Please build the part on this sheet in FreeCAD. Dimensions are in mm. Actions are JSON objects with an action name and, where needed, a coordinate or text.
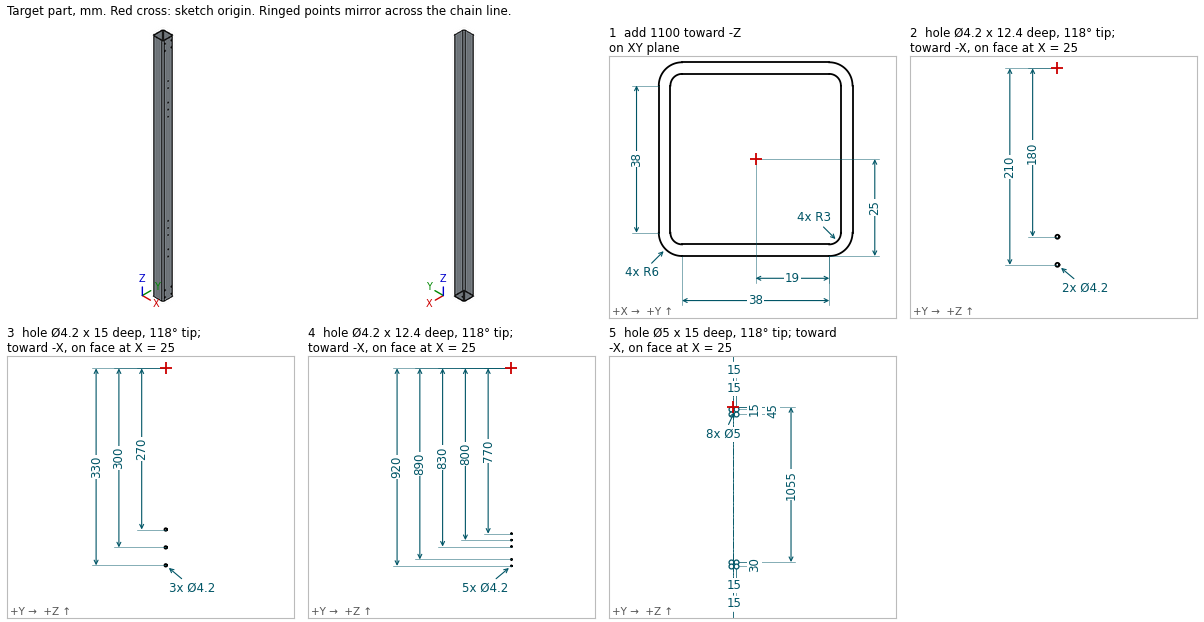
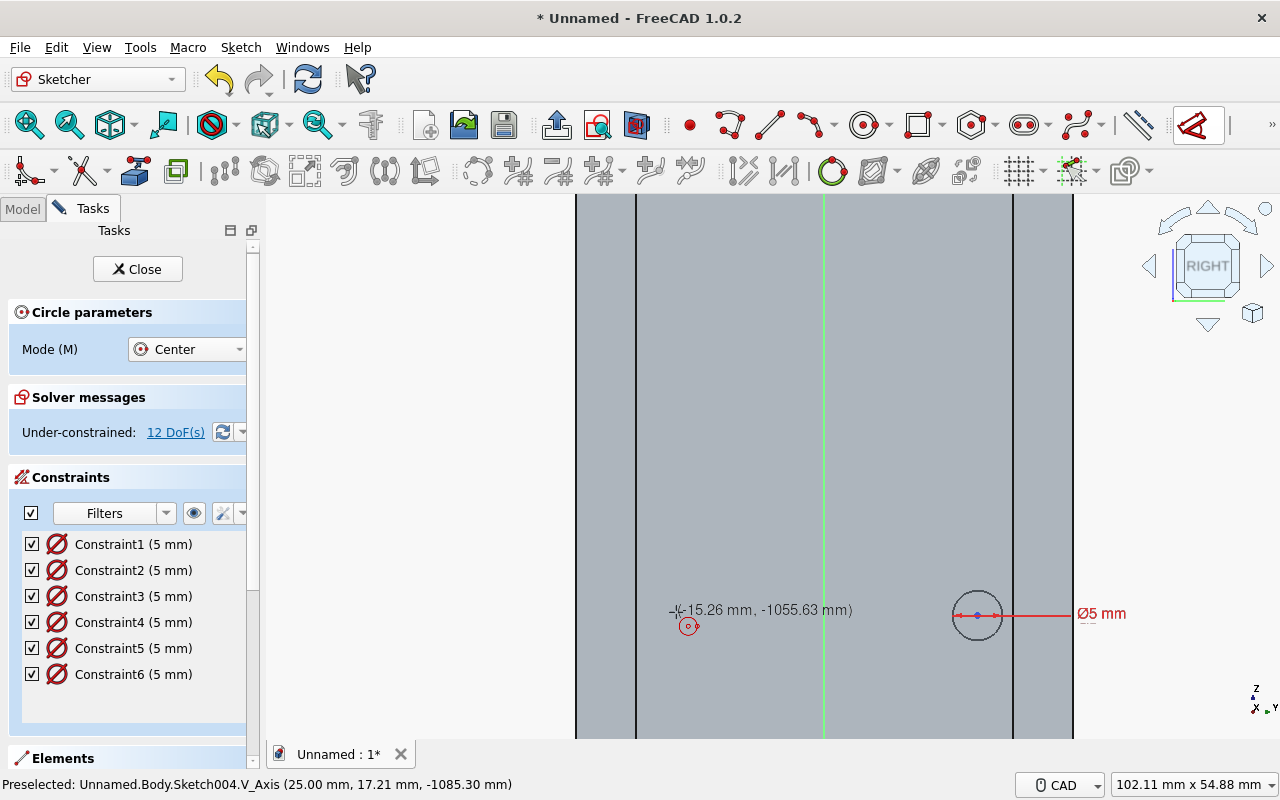
{"action": "scroll", "coordinate": [700, 637], "scroll_direction": "down", "scroll_amount": 17}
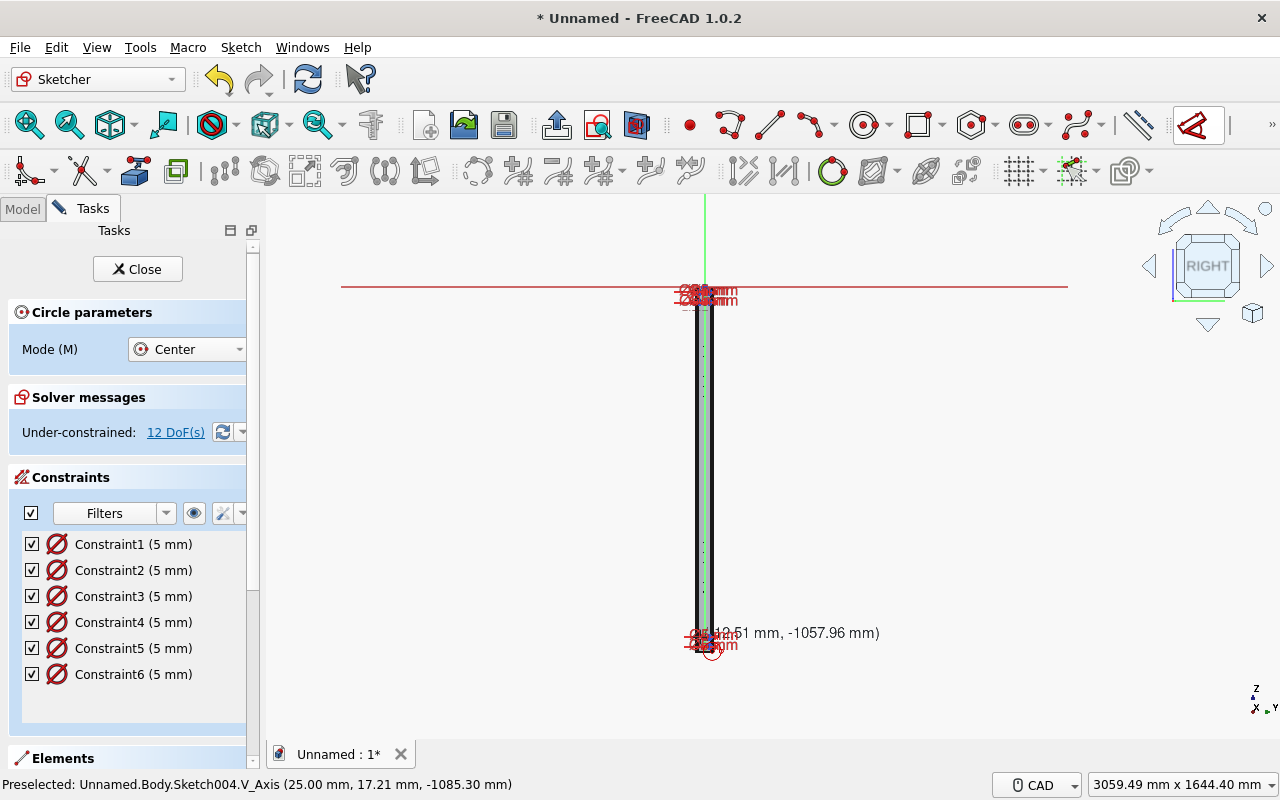
{"action": "scroll", "coordinate": [700, 637], "scroll_direction": "up", "scroll_amount": 6}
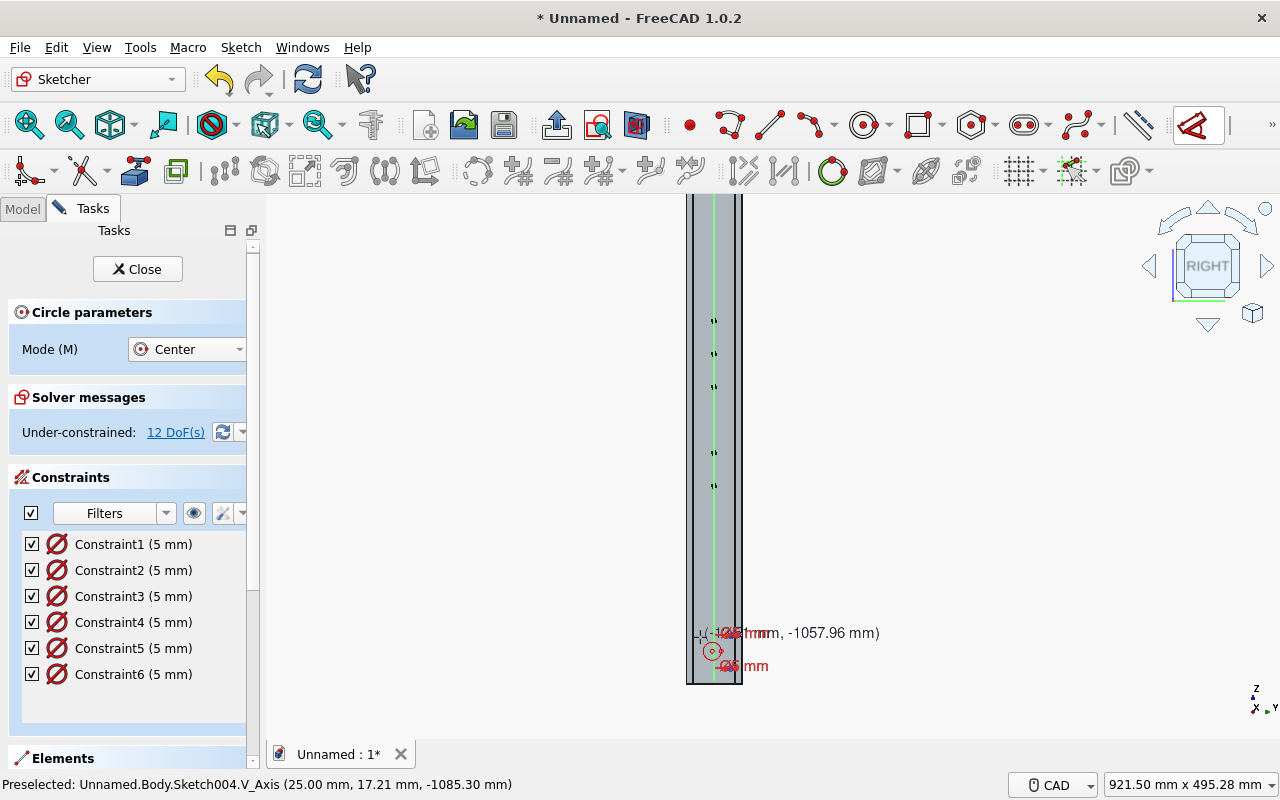
{"action": "left_click", "coordinate": [698, 635]}
{"action": "mouse_move", "coordinate": [700, 633]}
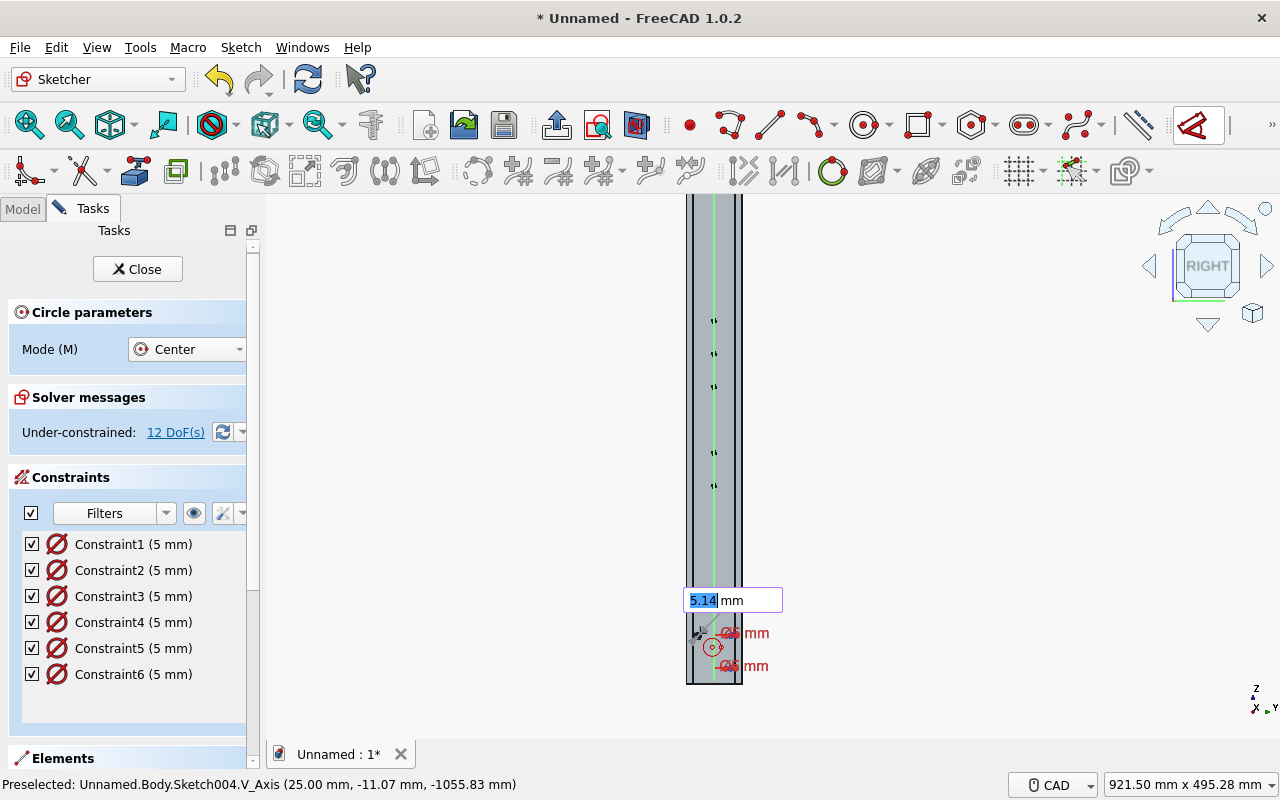
{"action": "type", "text": "5"}
{"action": "key", "text": "Return"}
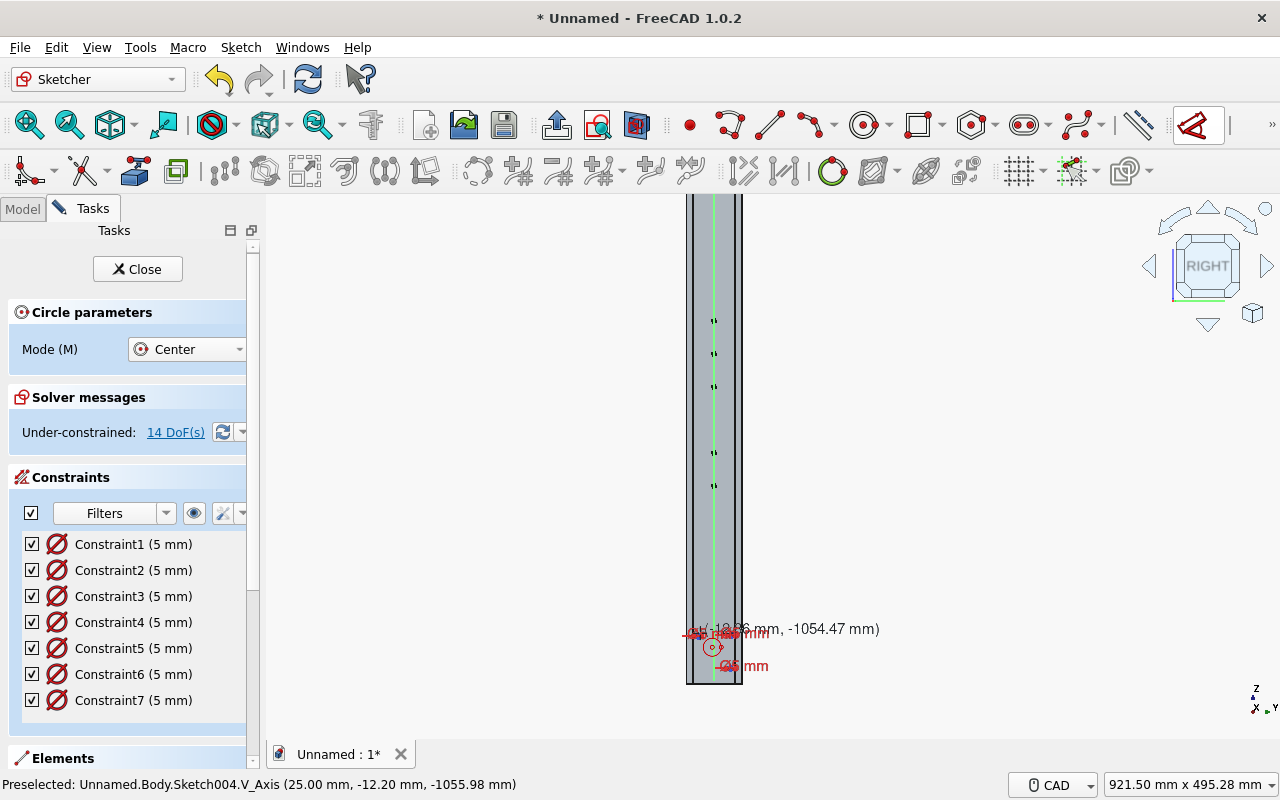
{"action": "scroll", "coordinate": [698, 668], "scroll_direction": "up", "scroll_amount": 11}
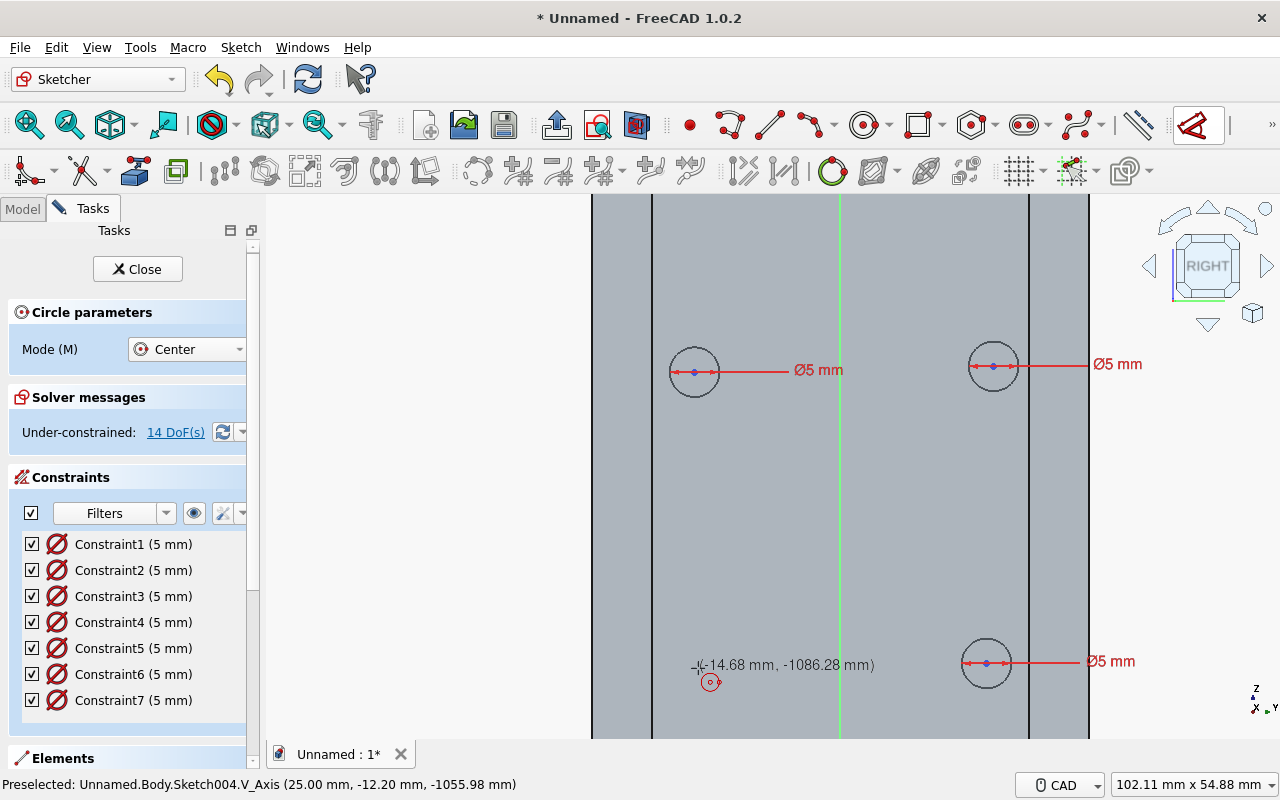
{"action": "scroll", "coordinate": [700, 645], "scroll_direction": "down", "scroll_amount": 17}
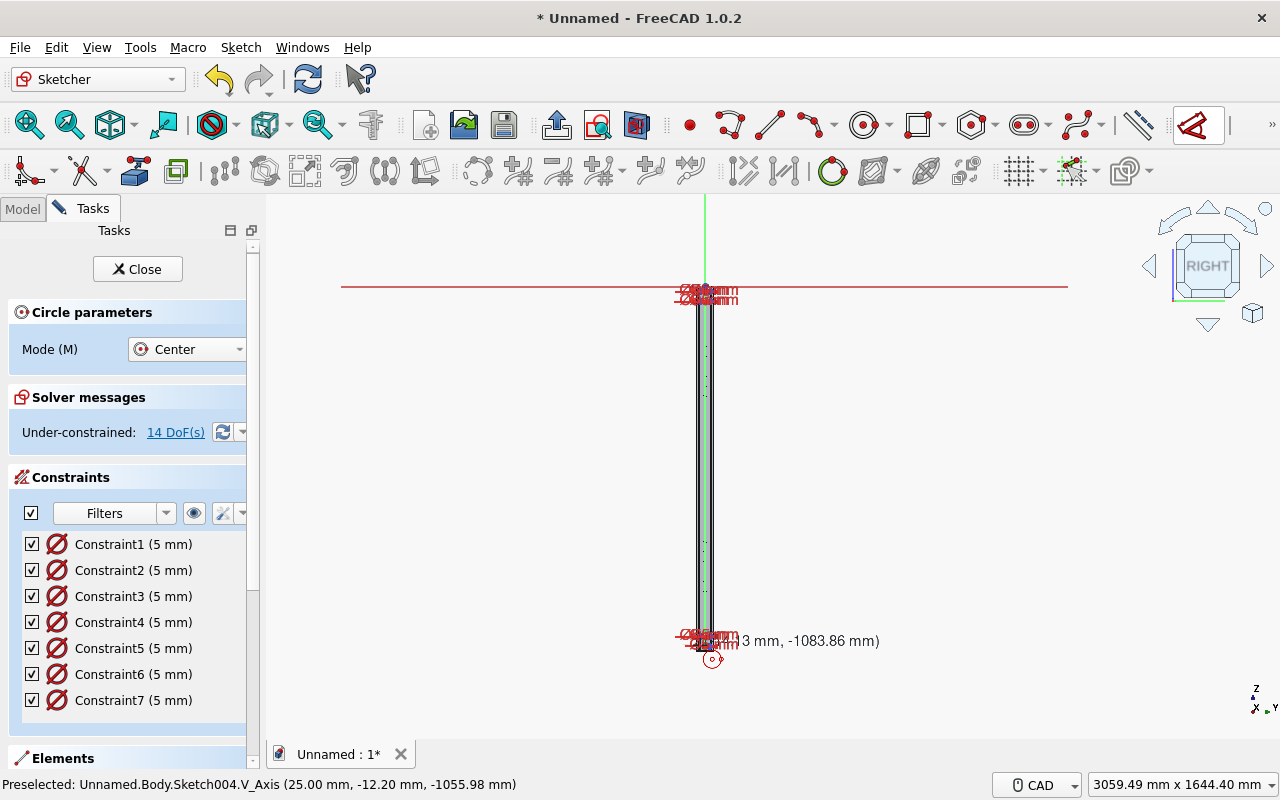
{"action": "scroll", "coordinate": [700, 646], "scroll_direction": "up", "scroll_amount": 6}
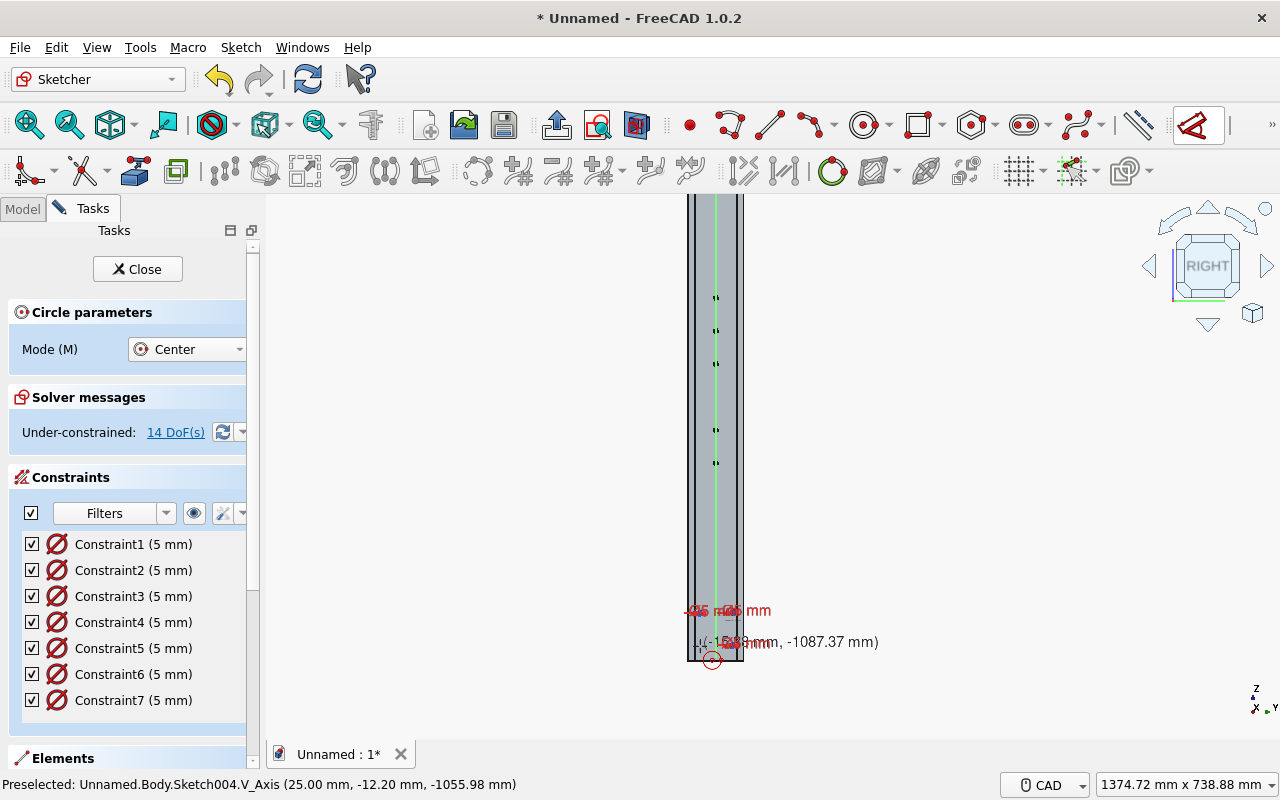
{"action": "left_click", "coordinate": [699, 645]}
{"action": "mouse_move", "coordinate": [701, 643]}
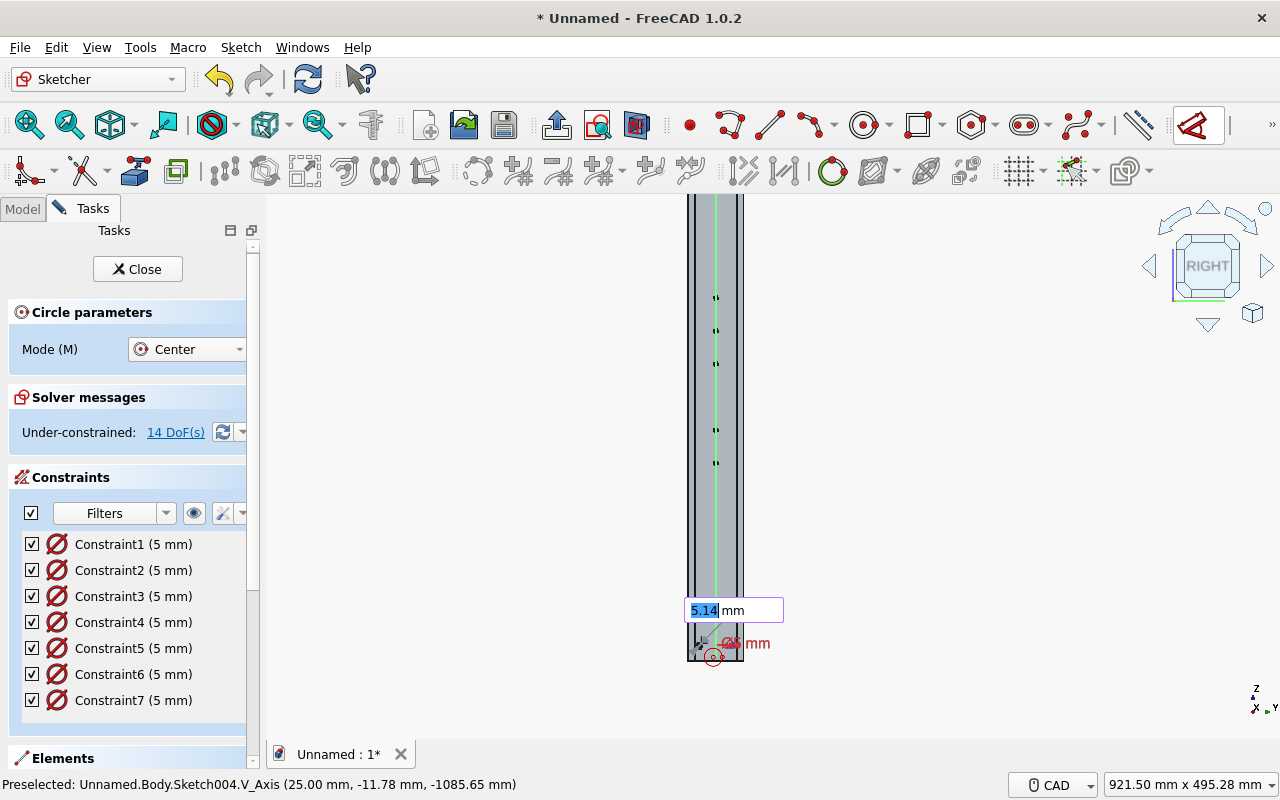
{"action": "type", "text": "5"}
{"action": "key", "text": "Return"}
{"action": "key", "text": "Escape"}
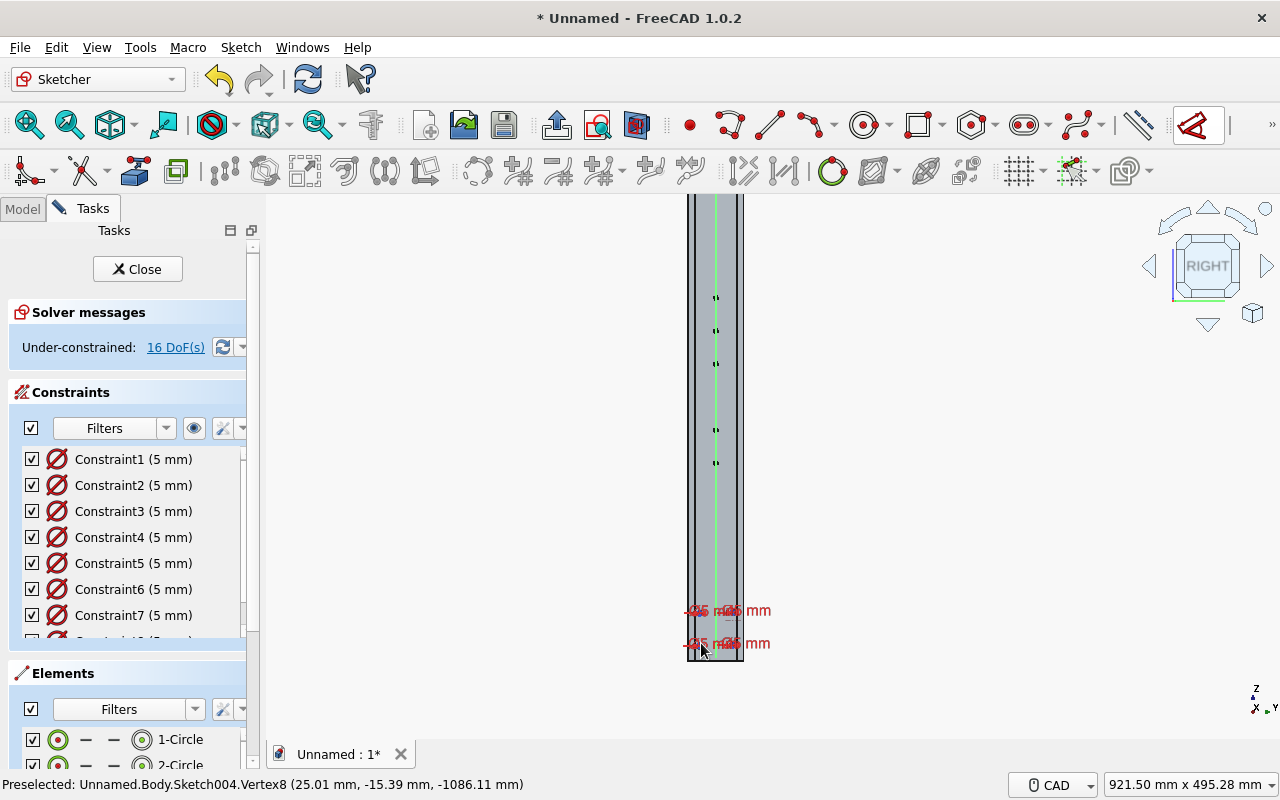
{"action": "scroll", "coordinate": [700, 646], "scroll_direction": "down", "scroll_amount": 6}